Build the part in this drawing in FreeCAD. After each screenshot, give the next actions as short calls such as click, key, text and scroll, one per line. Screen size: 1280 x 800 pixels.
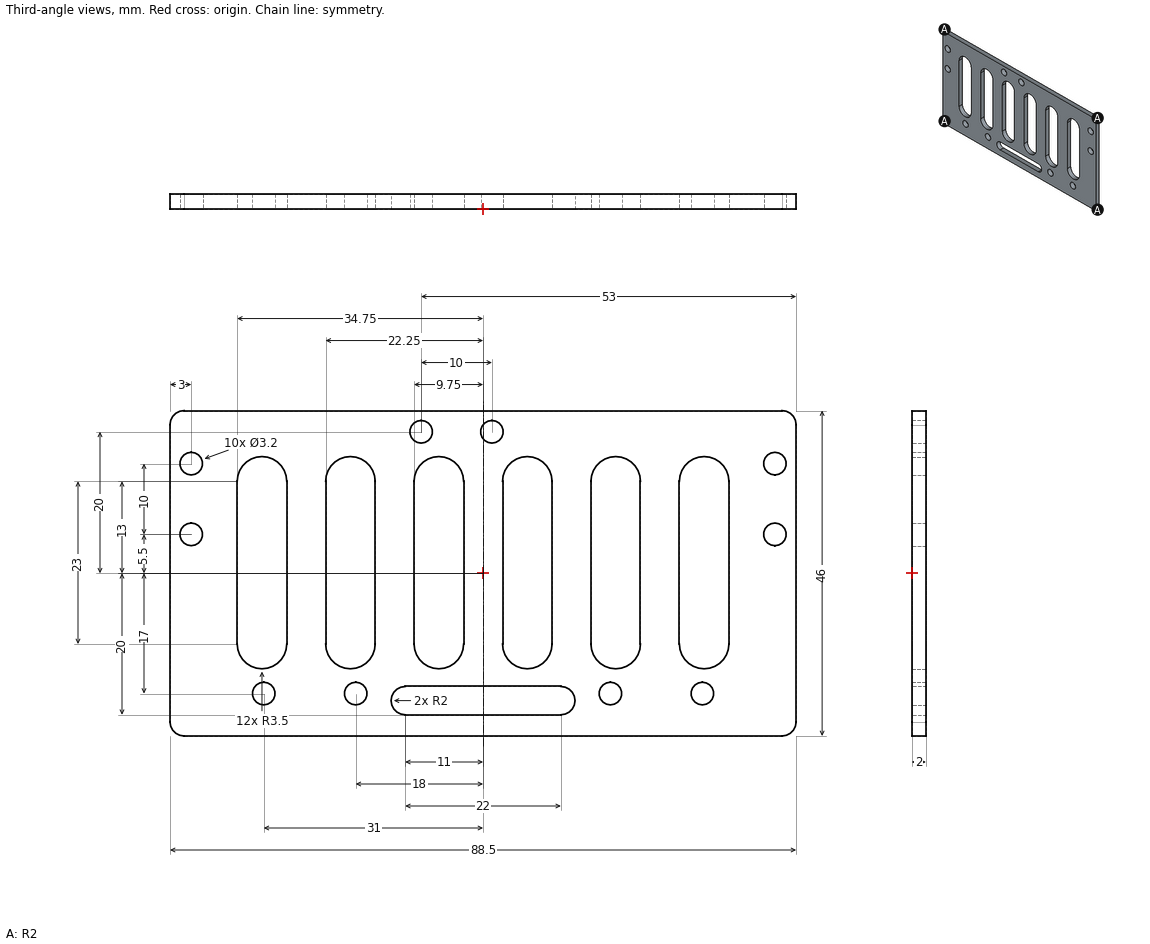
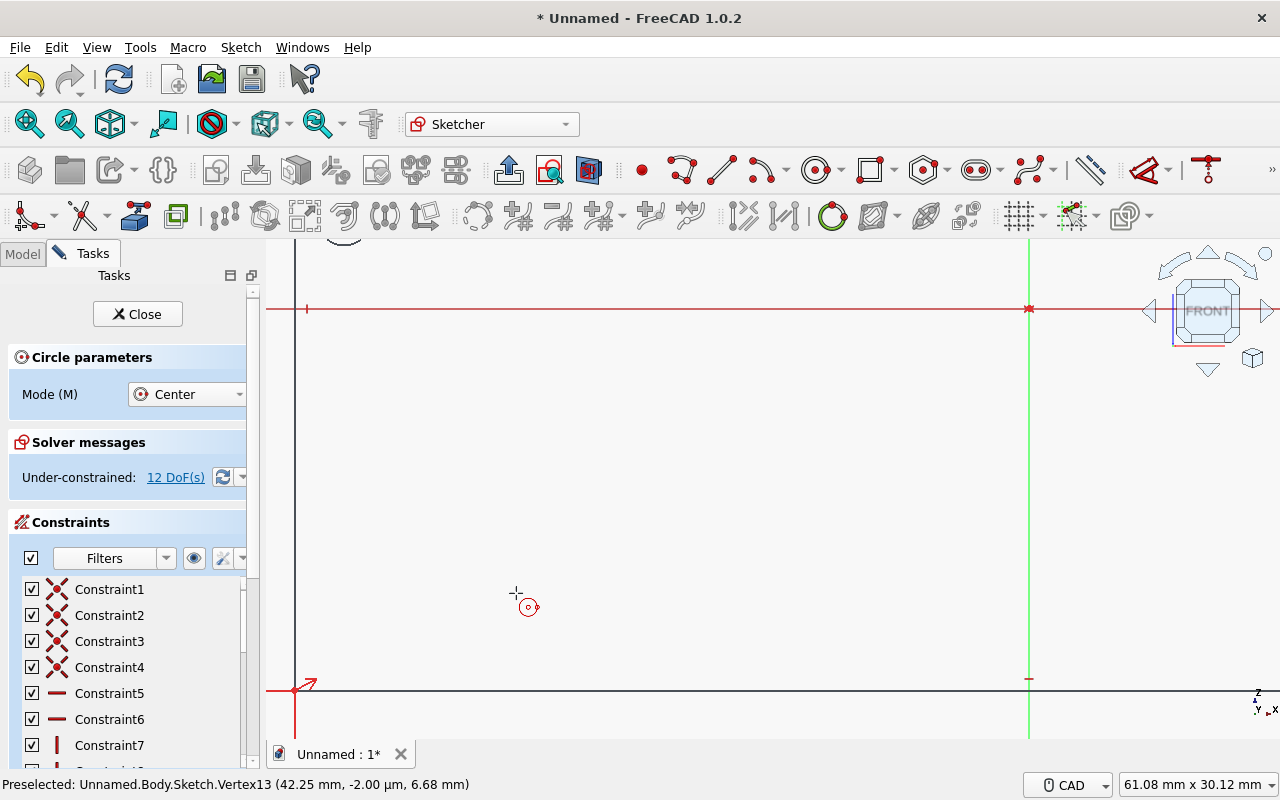
click(514, 591)
move(533, 572)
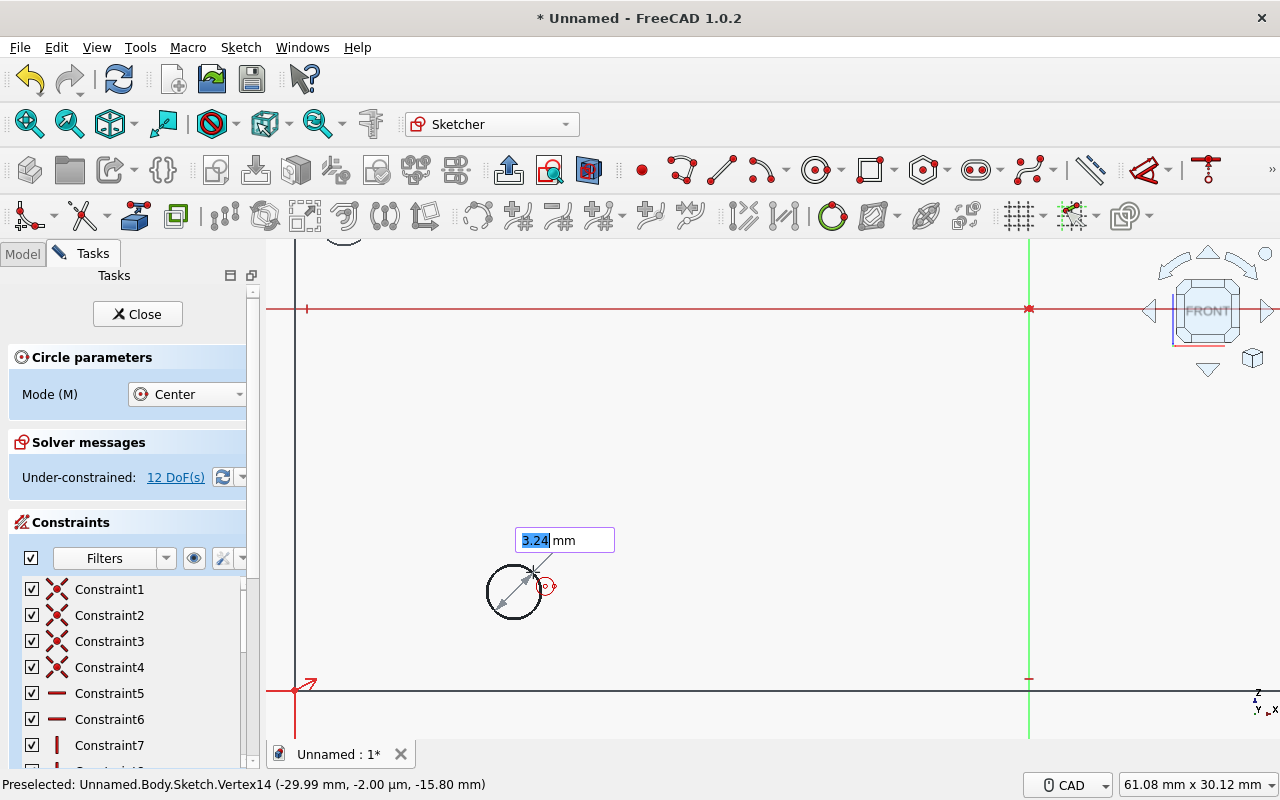
text(3.2)
key(Return)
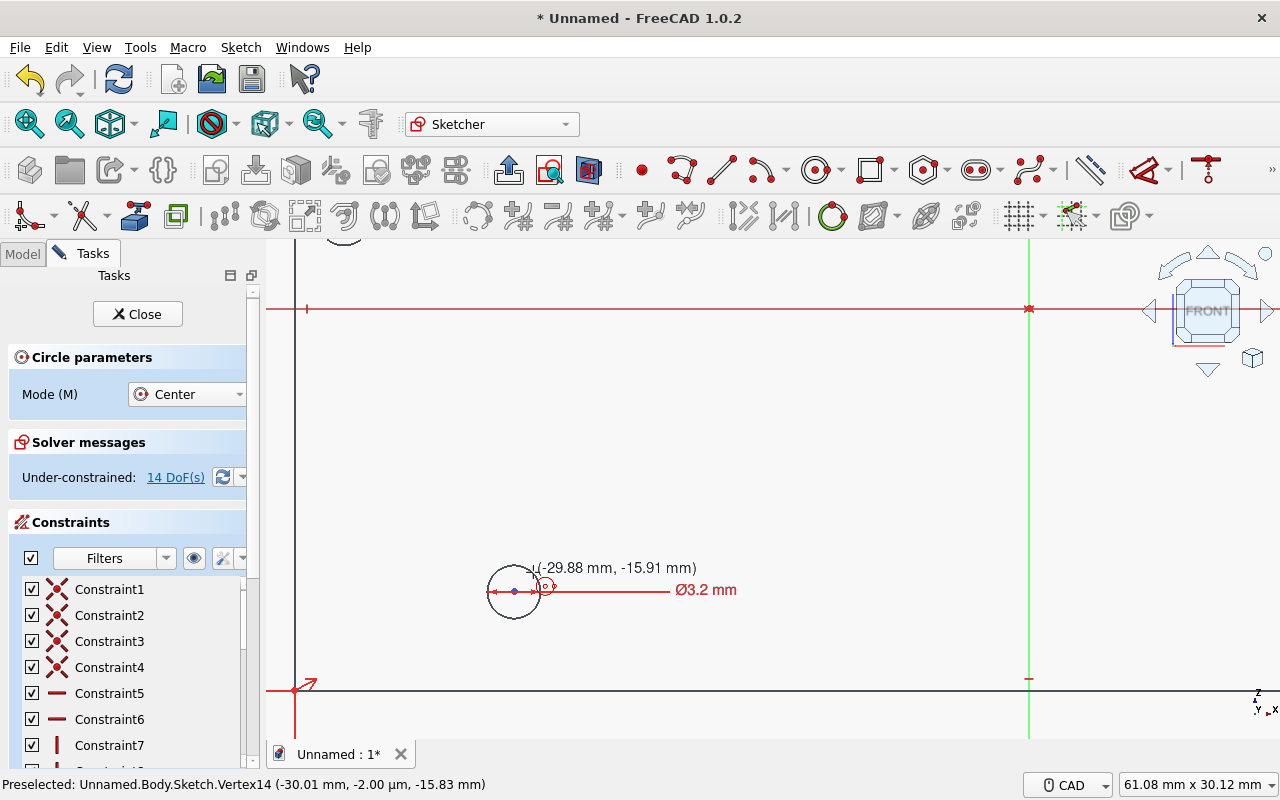
click(730, 591)
move(749, 572)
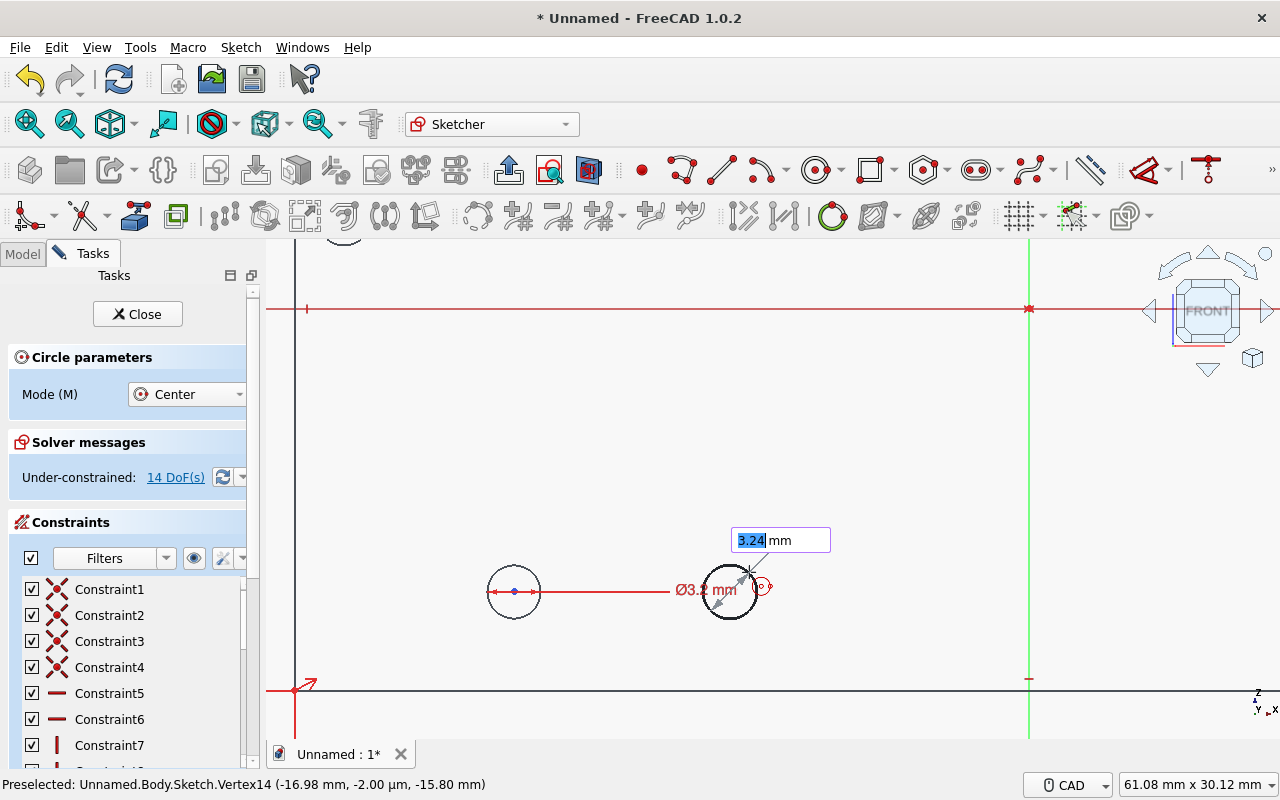
text(3.2)
key(Return)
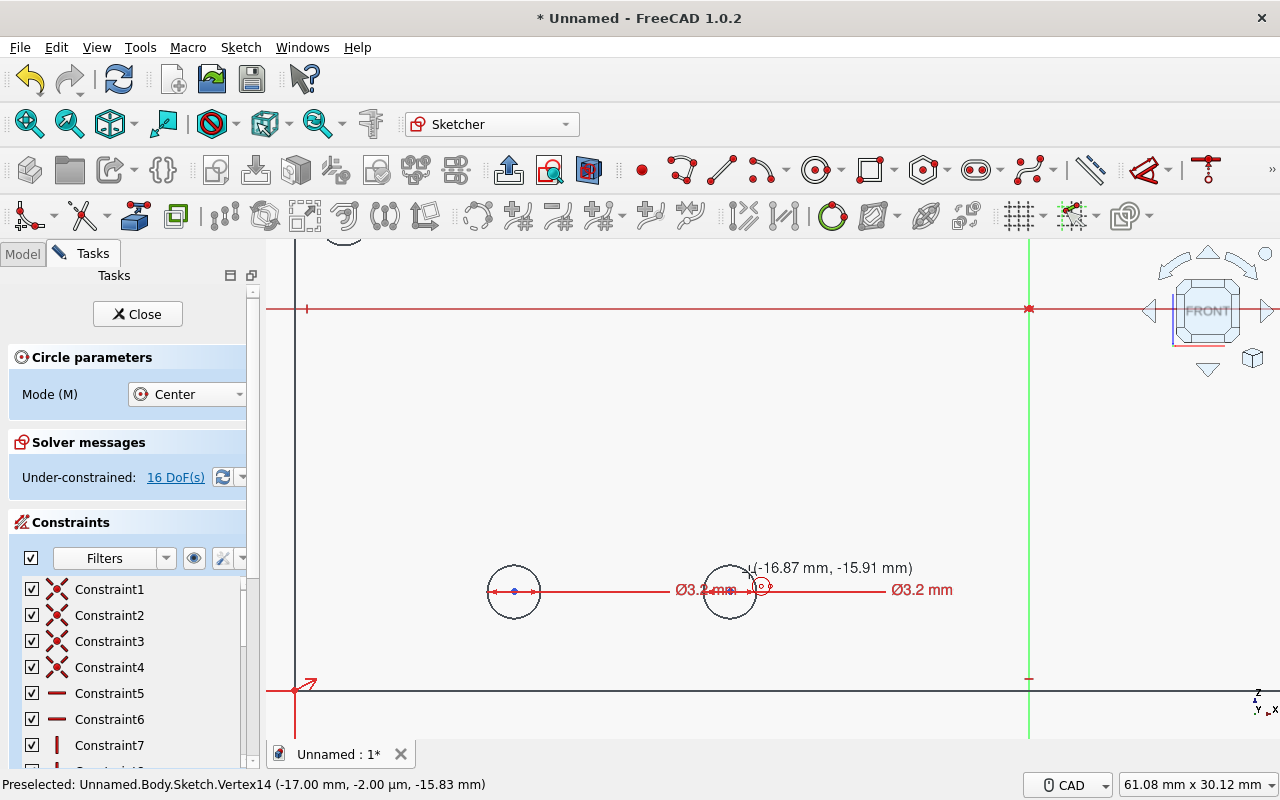
scroll(516, 594, down, 5)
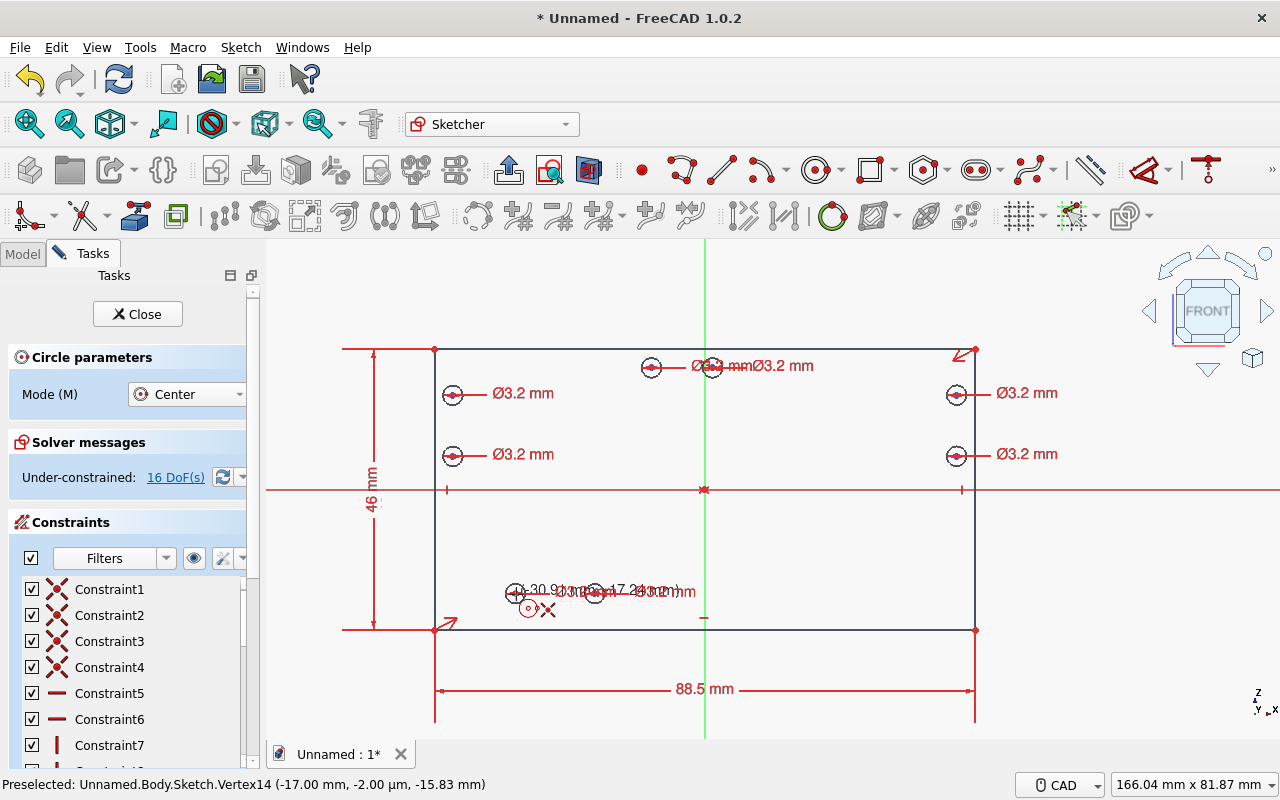
scroll(815, 593, up, 5)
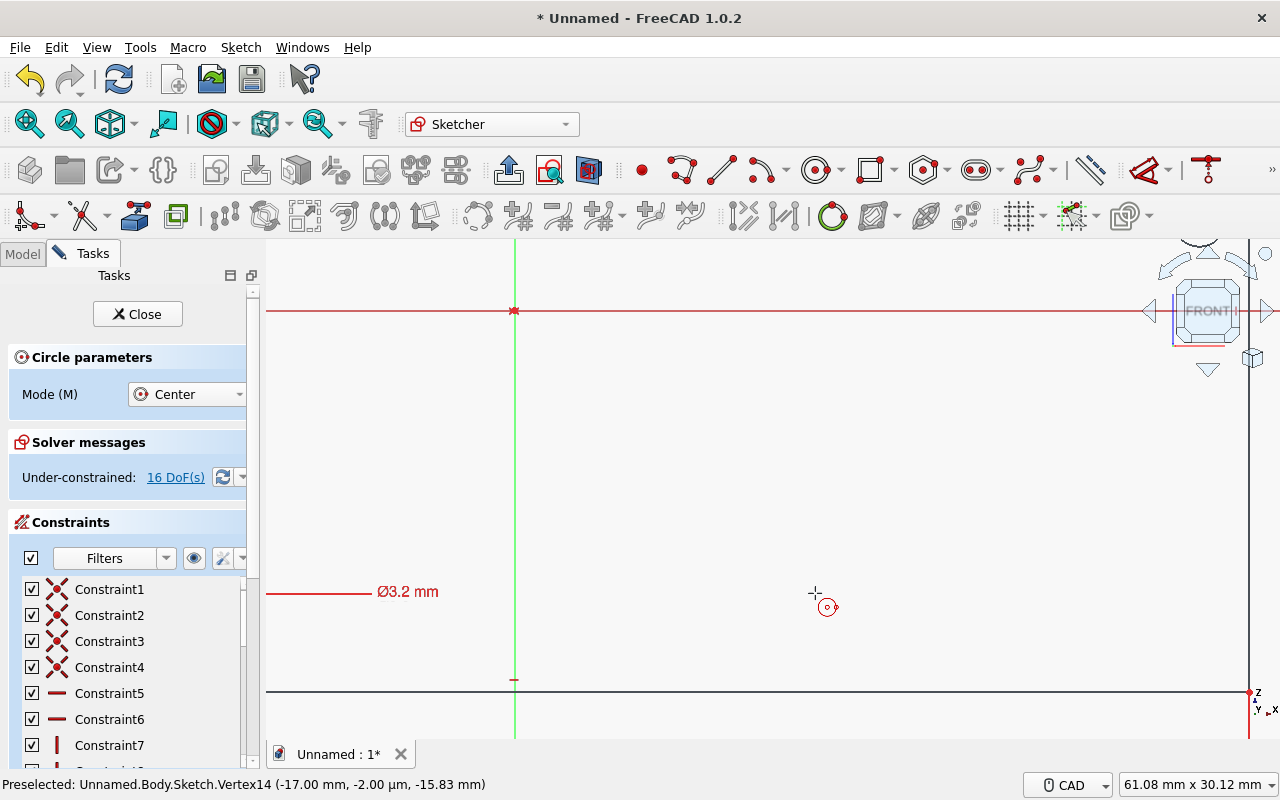
click(814, 593)
move(832, 574)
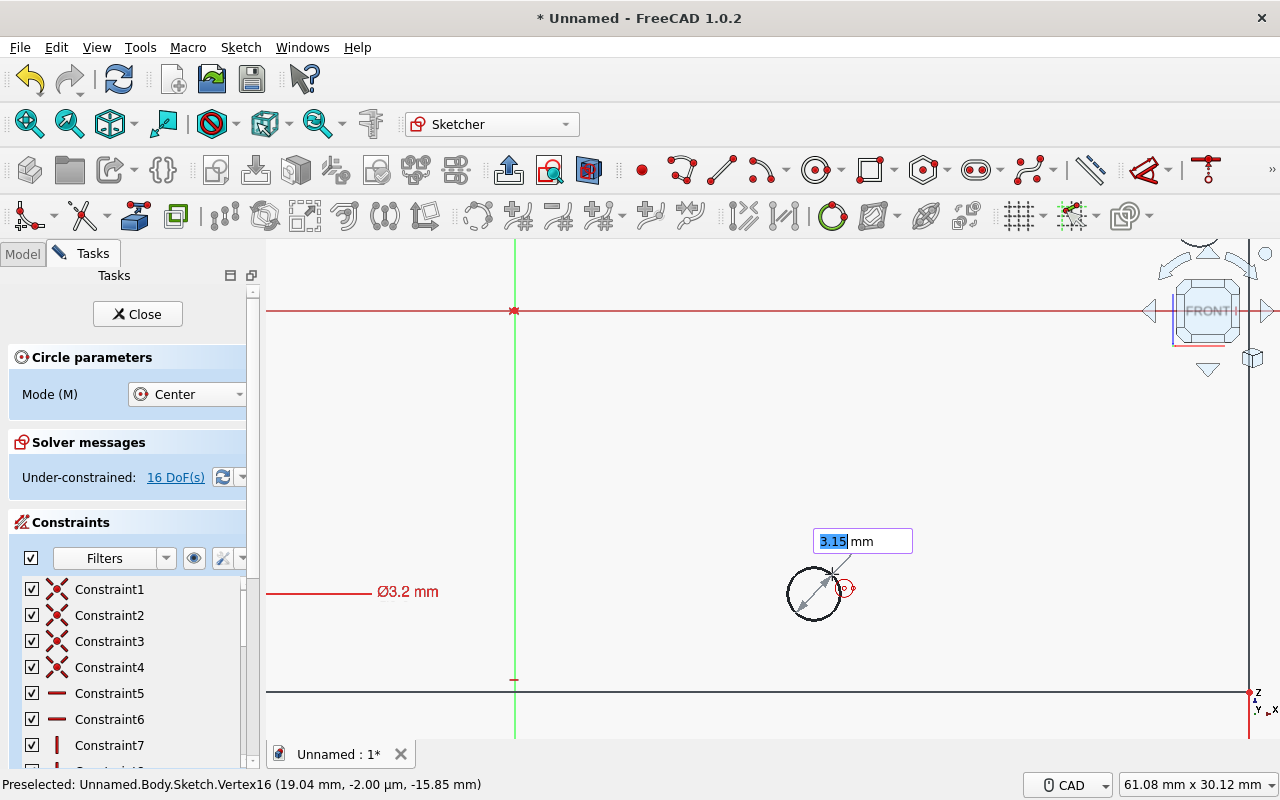
text(3.2)
key(Return)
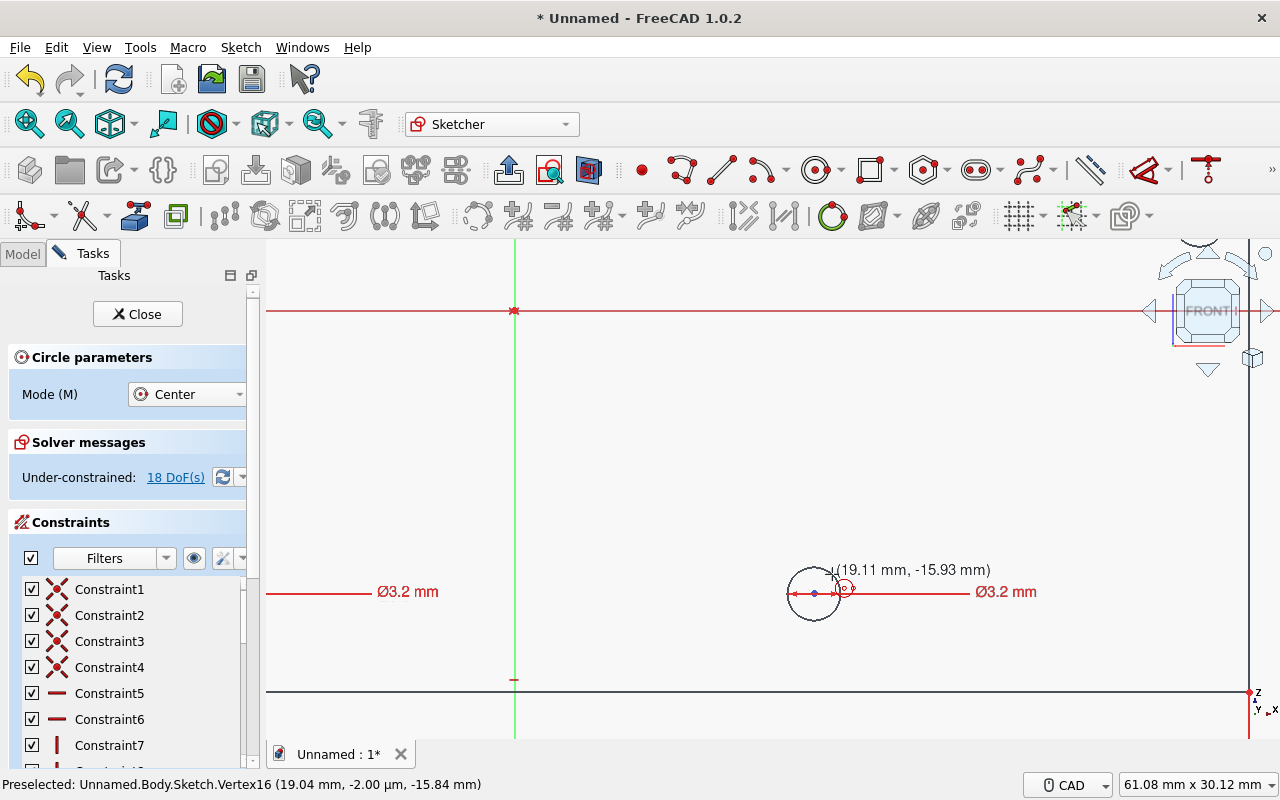
click(1029, 593)
move(1048, 574)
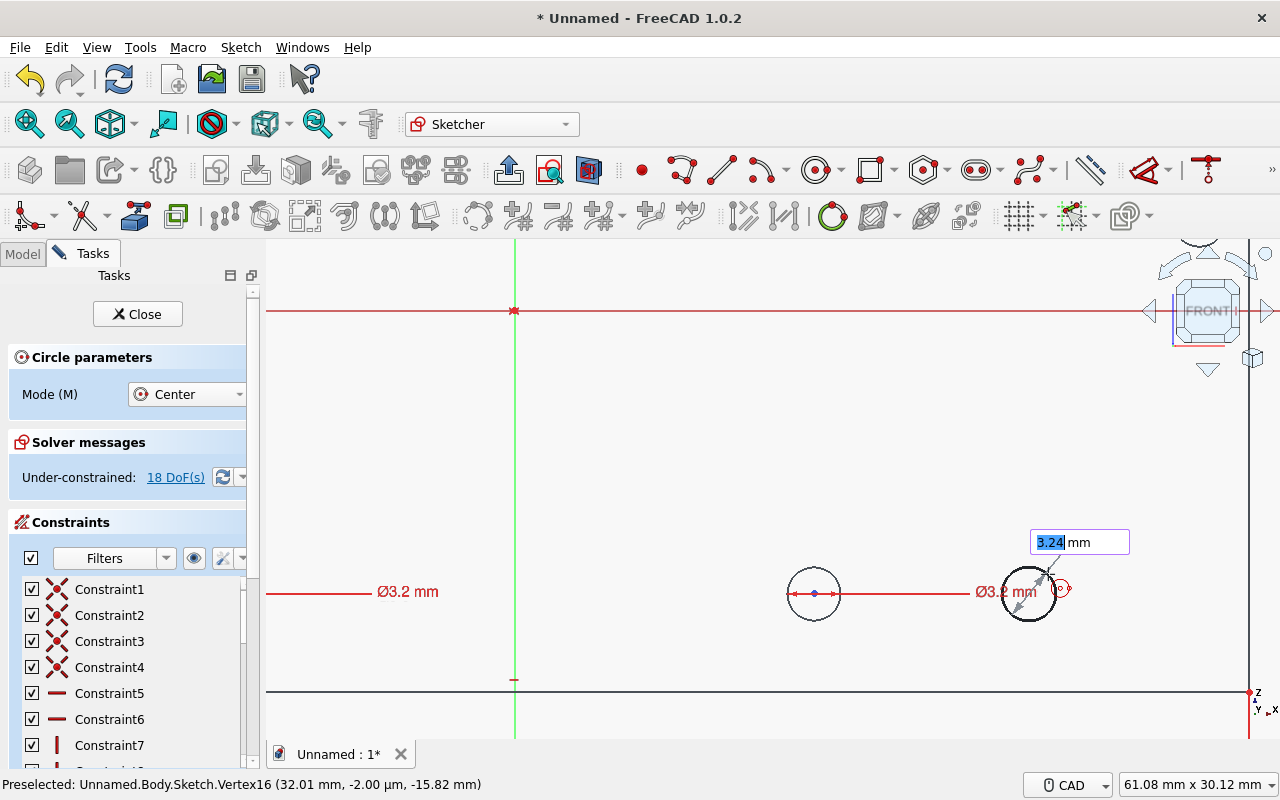
text(3.2)
key(Return)
key(Escape)